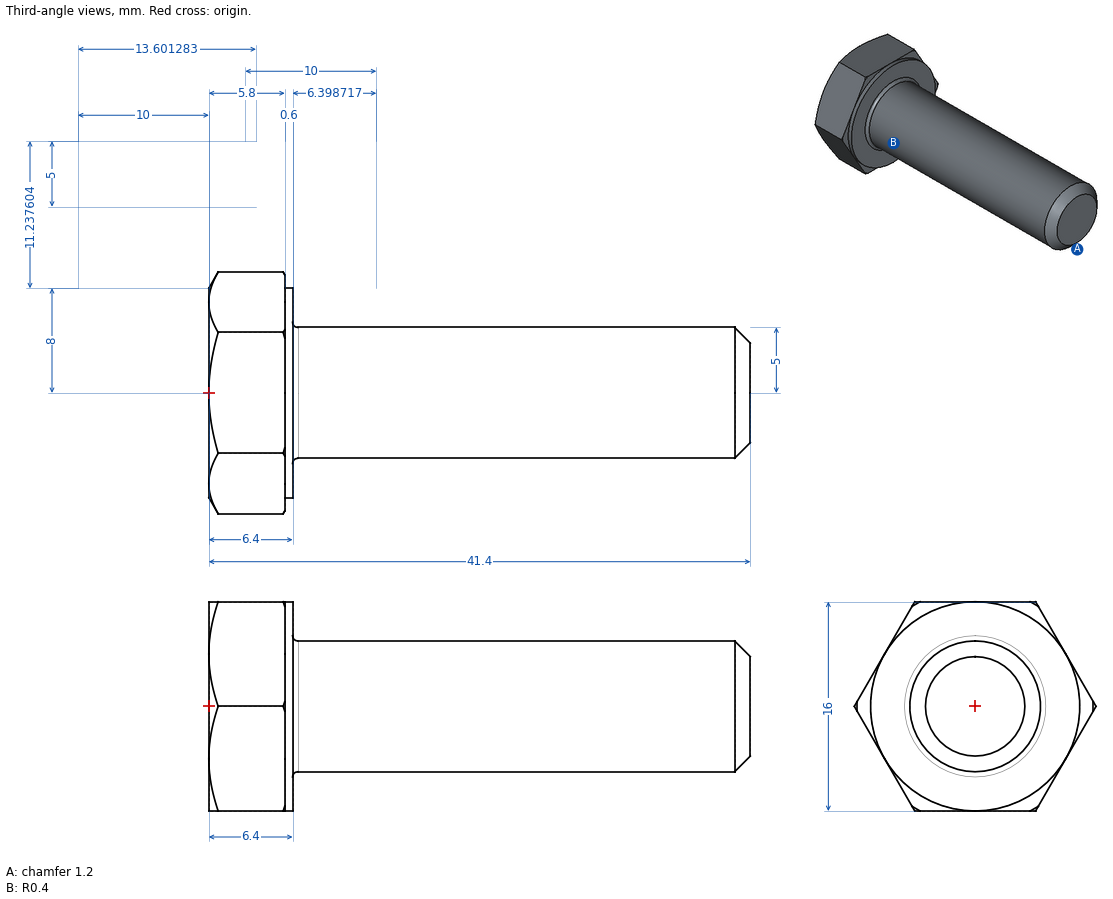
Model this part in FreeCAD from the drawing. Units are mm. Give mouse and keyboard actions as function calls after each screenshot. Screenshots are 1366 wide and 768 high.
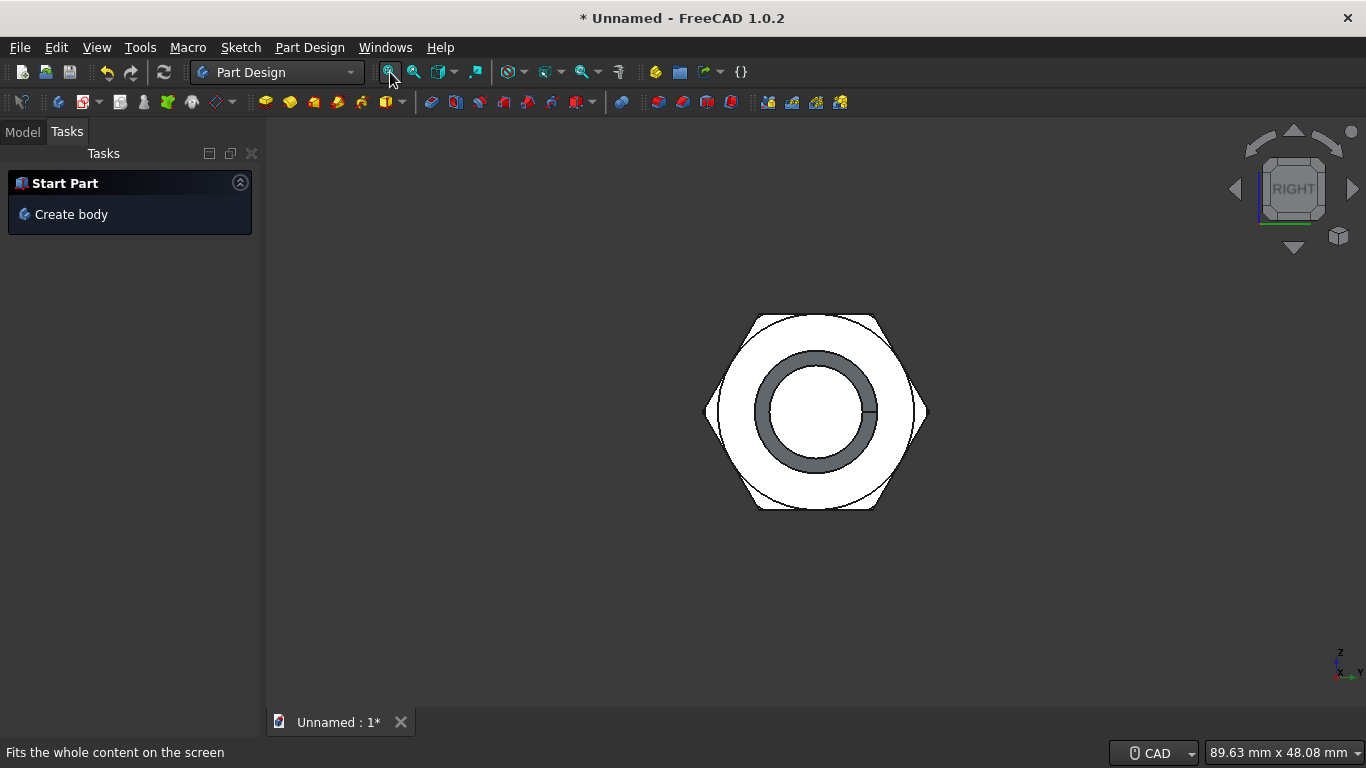
key(5)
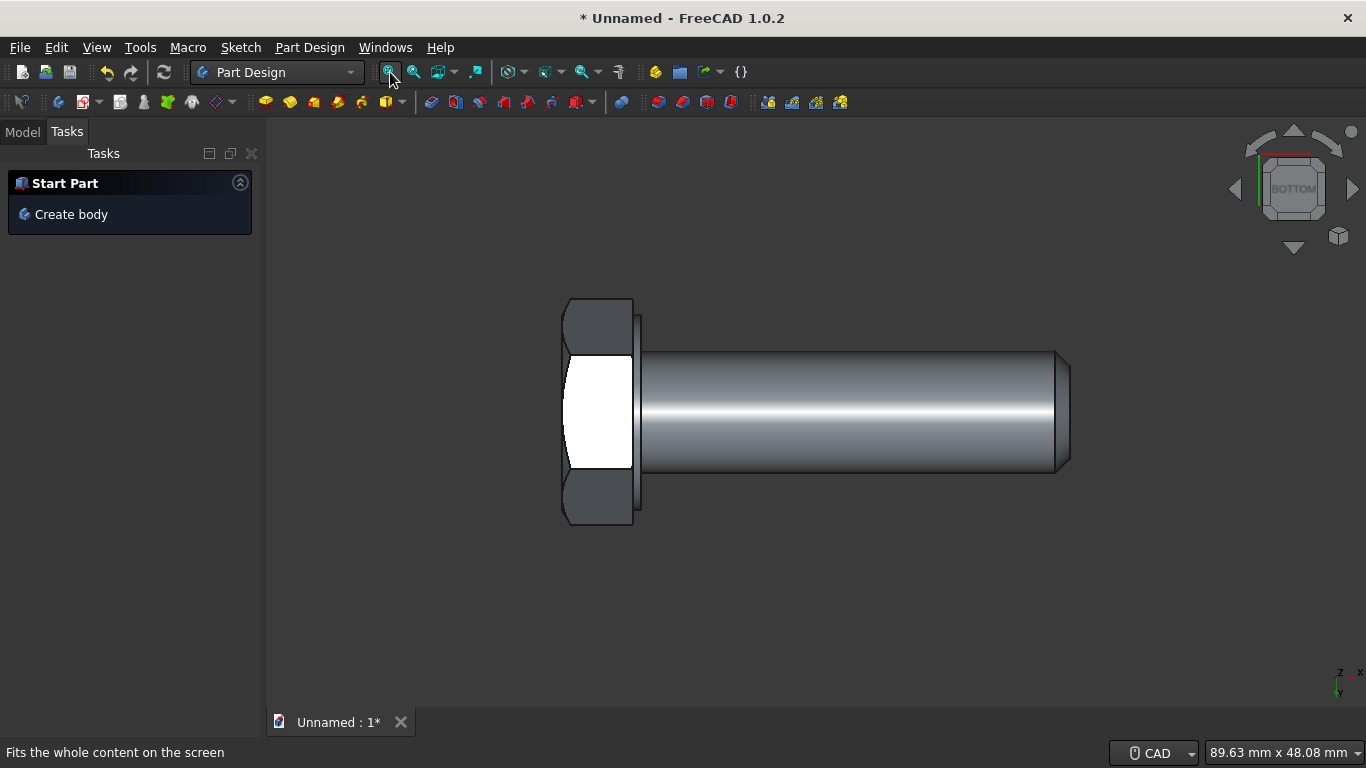
key(4)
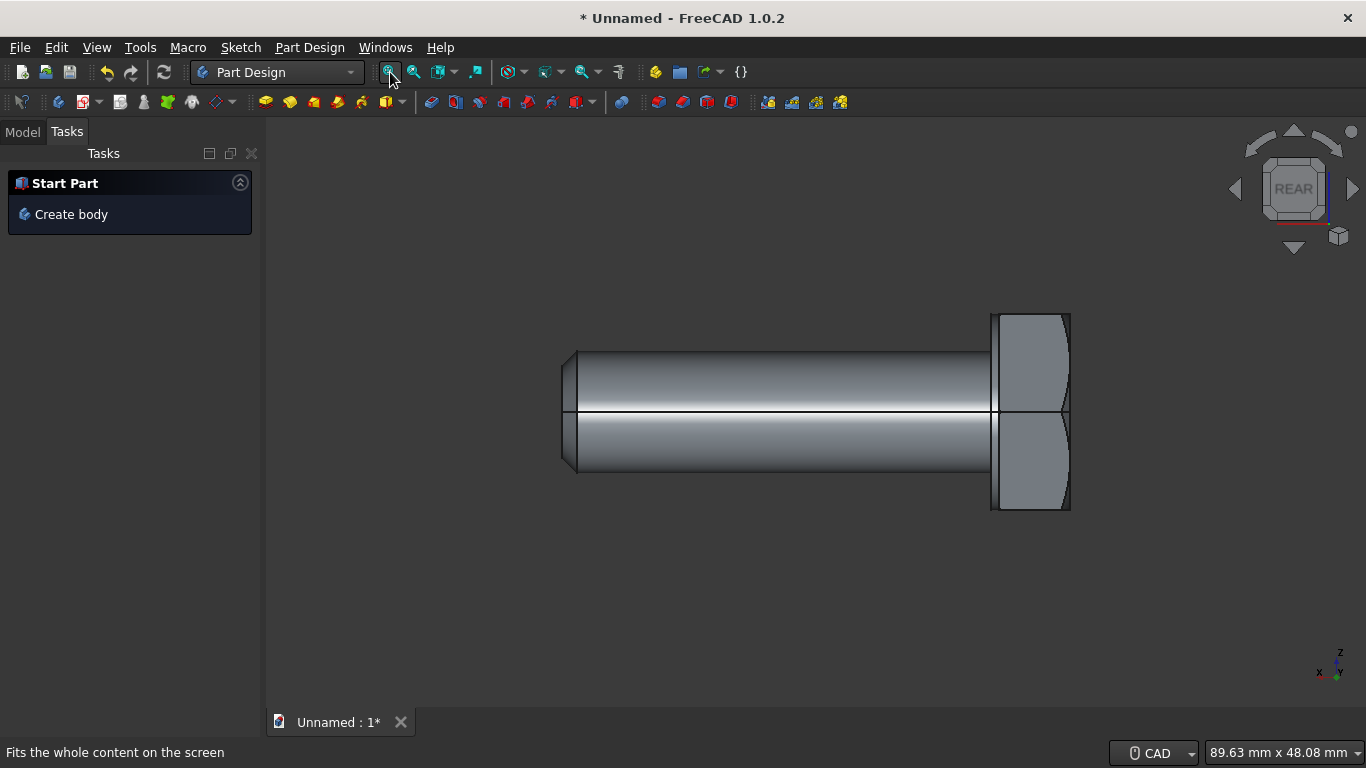
key(6)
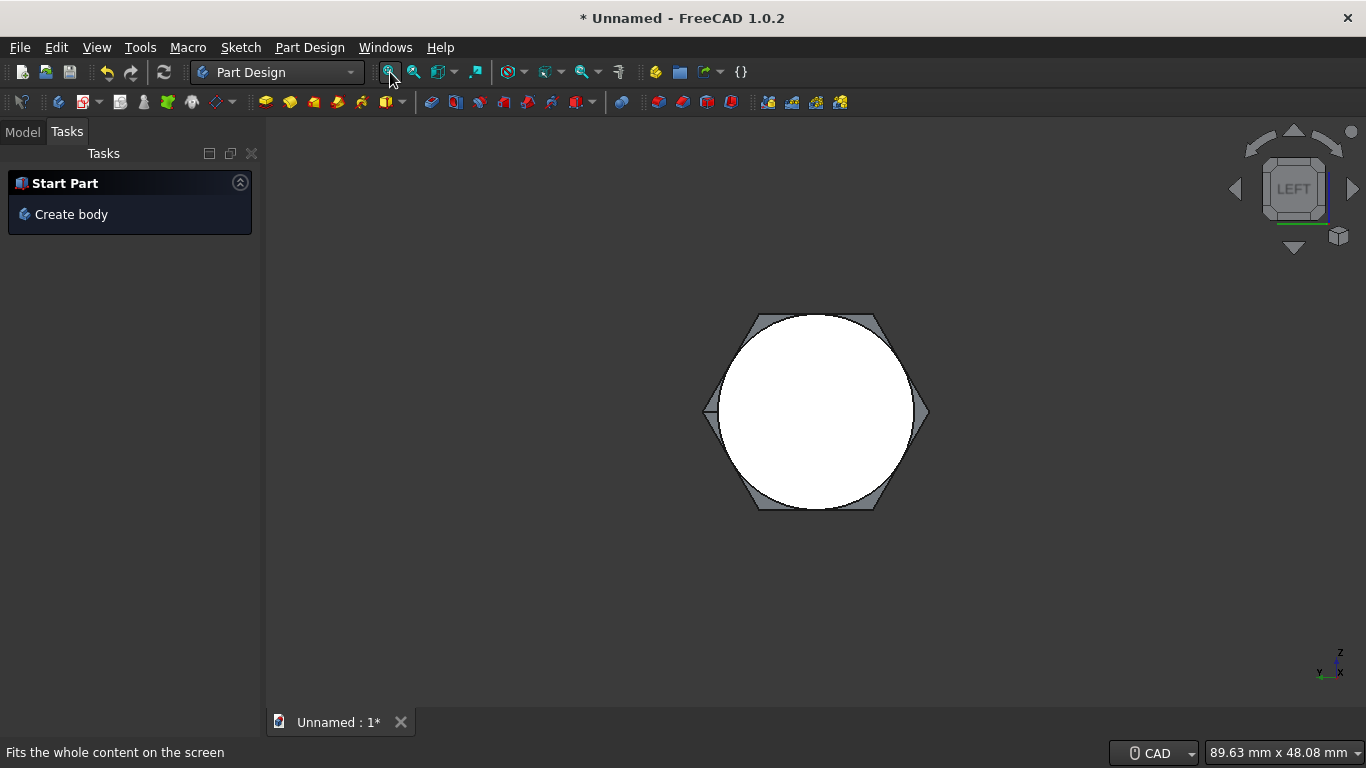
click(390, 72)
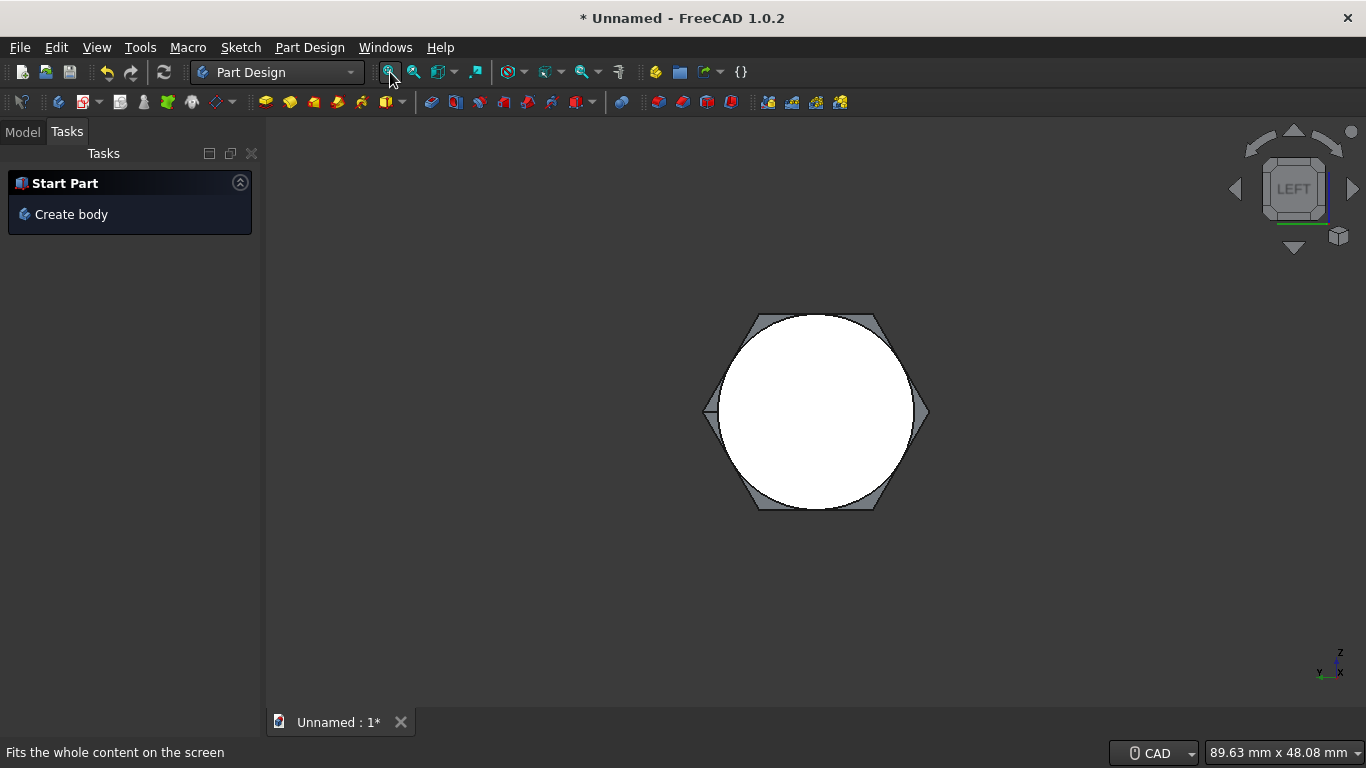
key(v)
key(3)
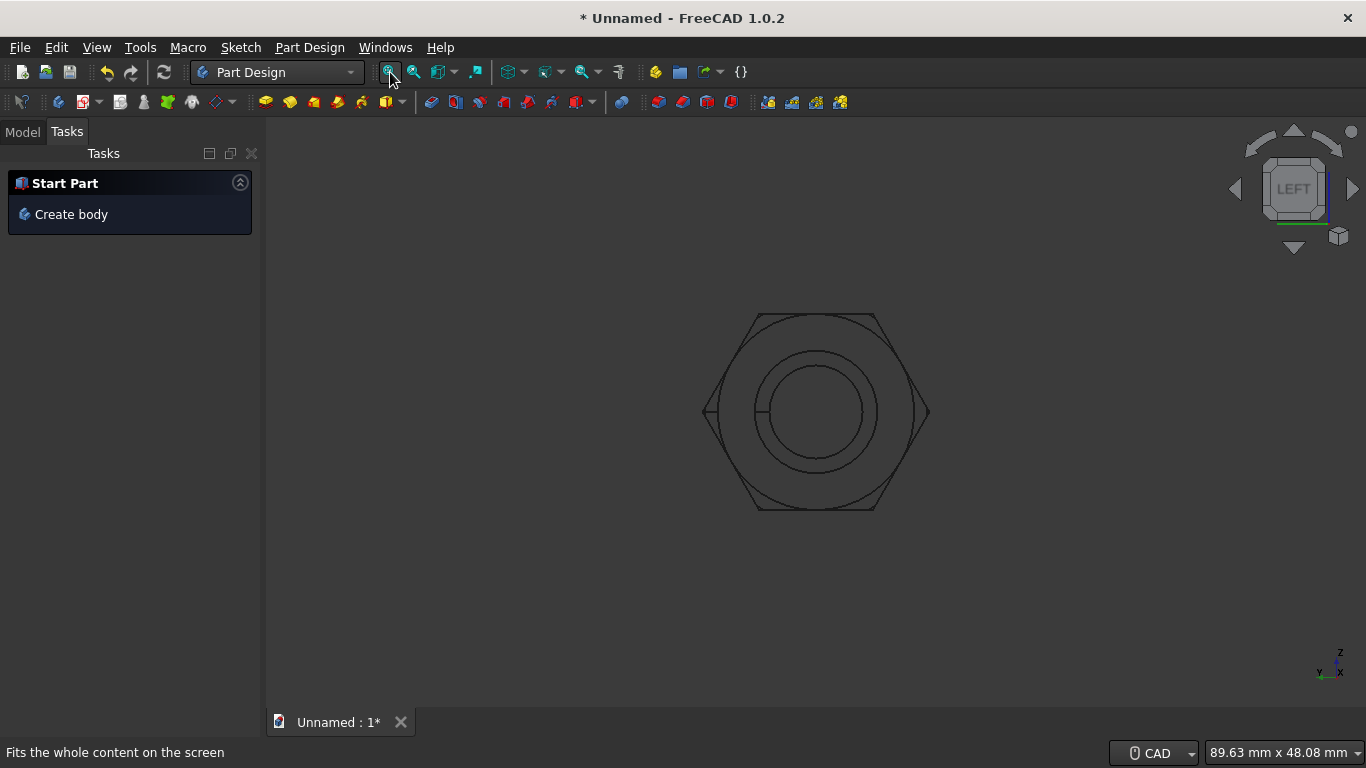
key(0)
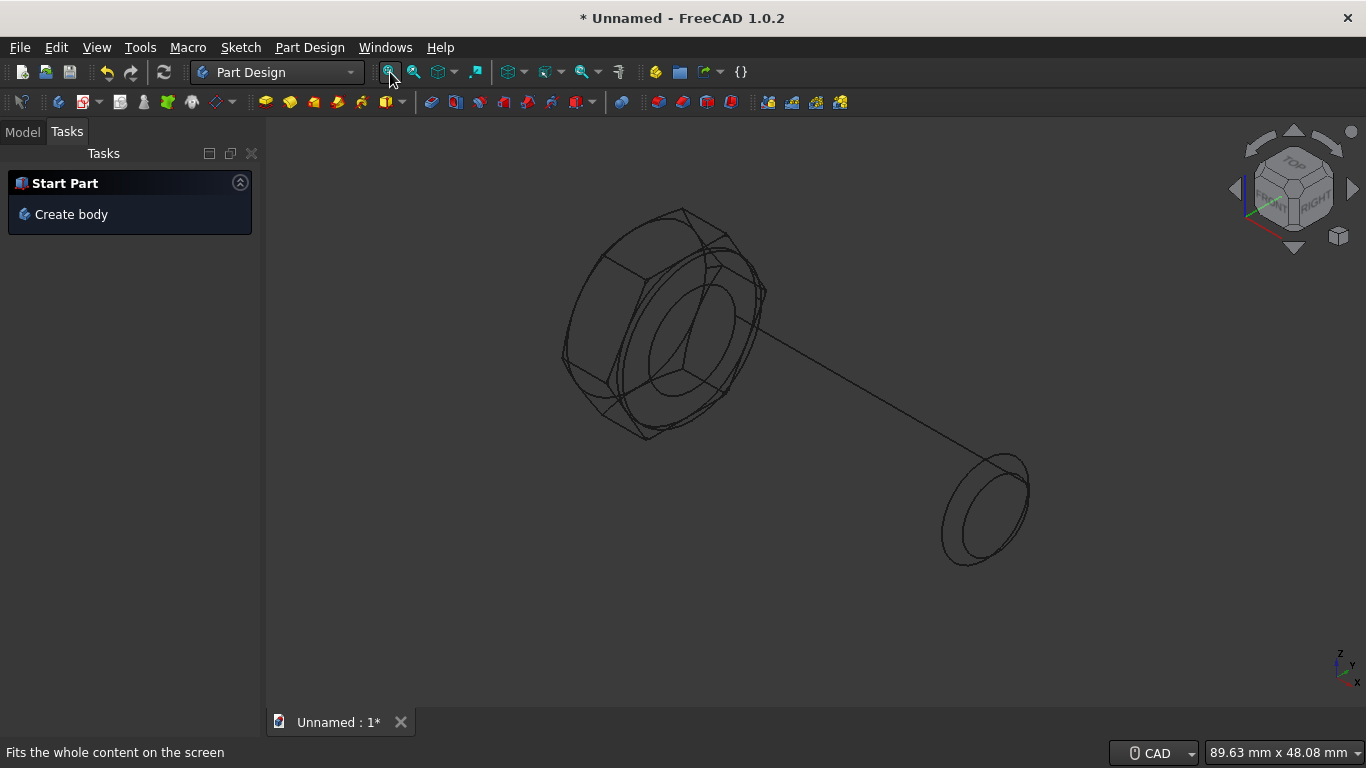
click(649, 364)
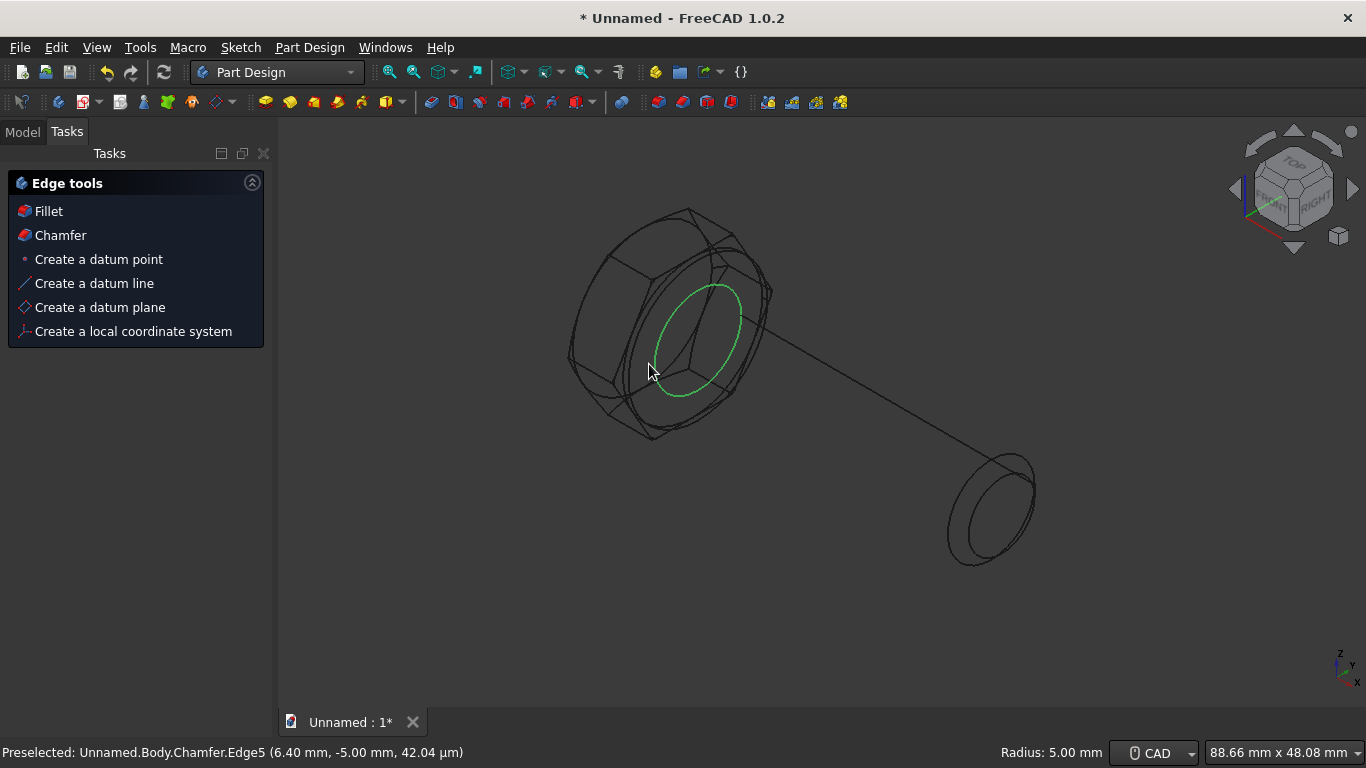
key(v)
key(1)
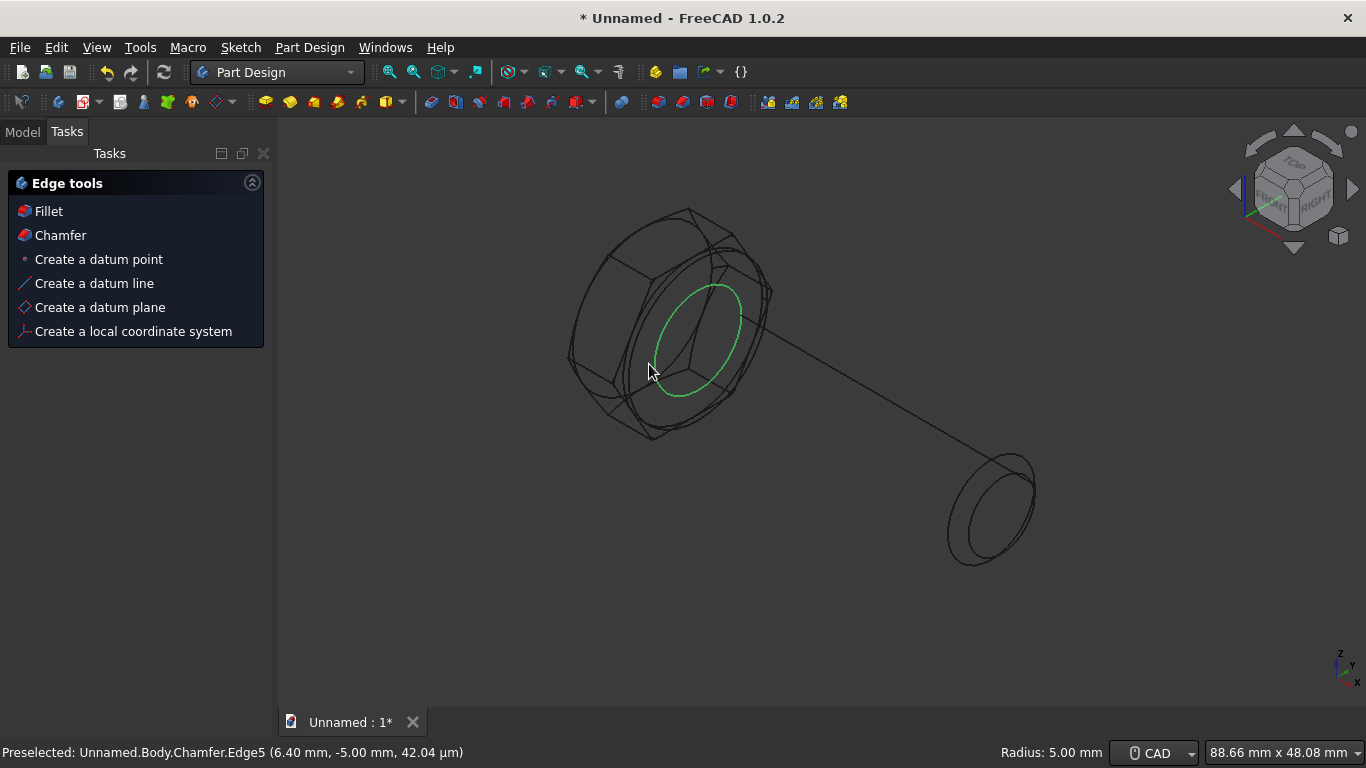
click(660, 102)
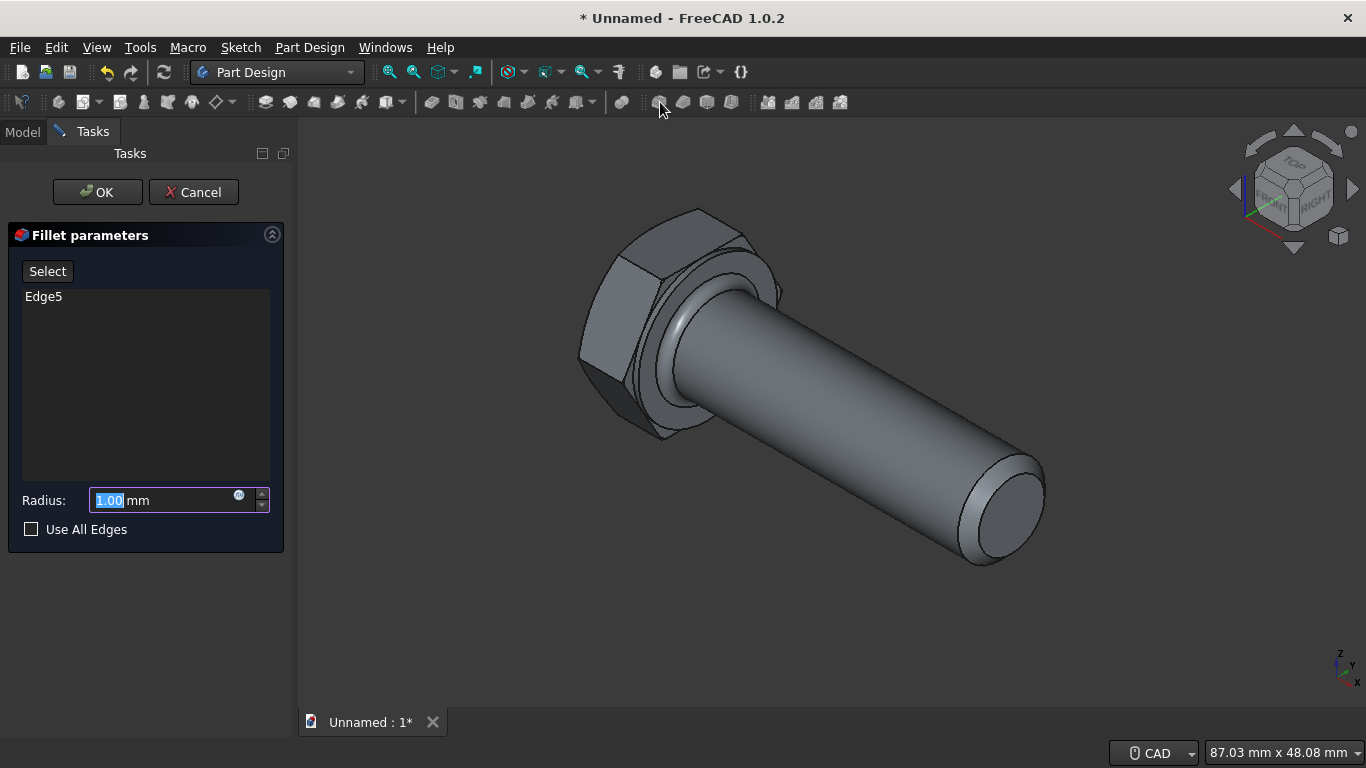
text(0.4)
key(Tab)